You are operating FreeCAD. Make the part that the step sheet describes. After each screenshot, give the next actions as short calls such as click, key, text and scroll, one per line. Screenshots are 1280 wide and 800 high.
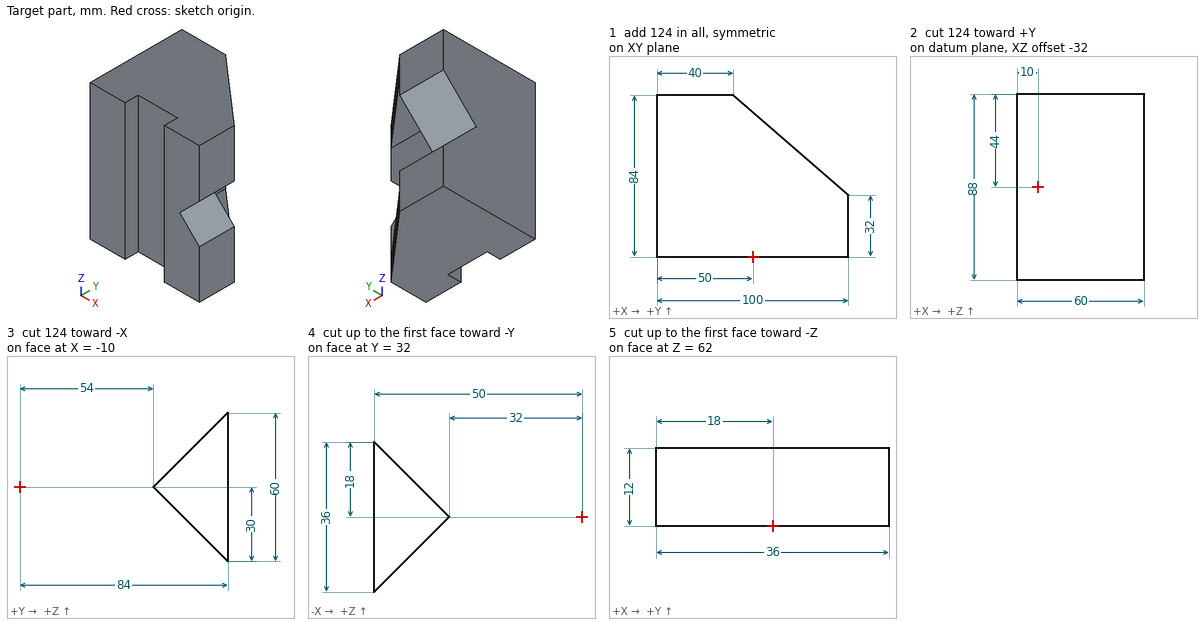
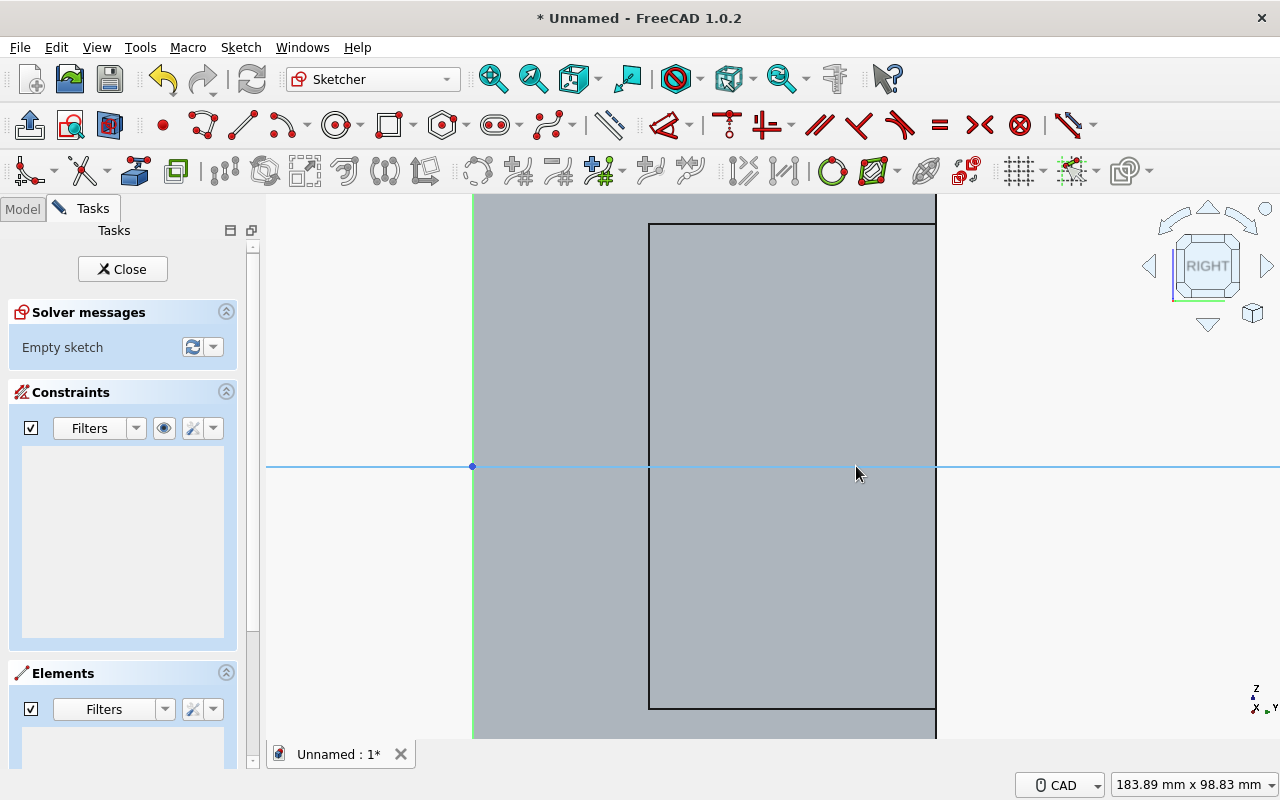
click(204, 126)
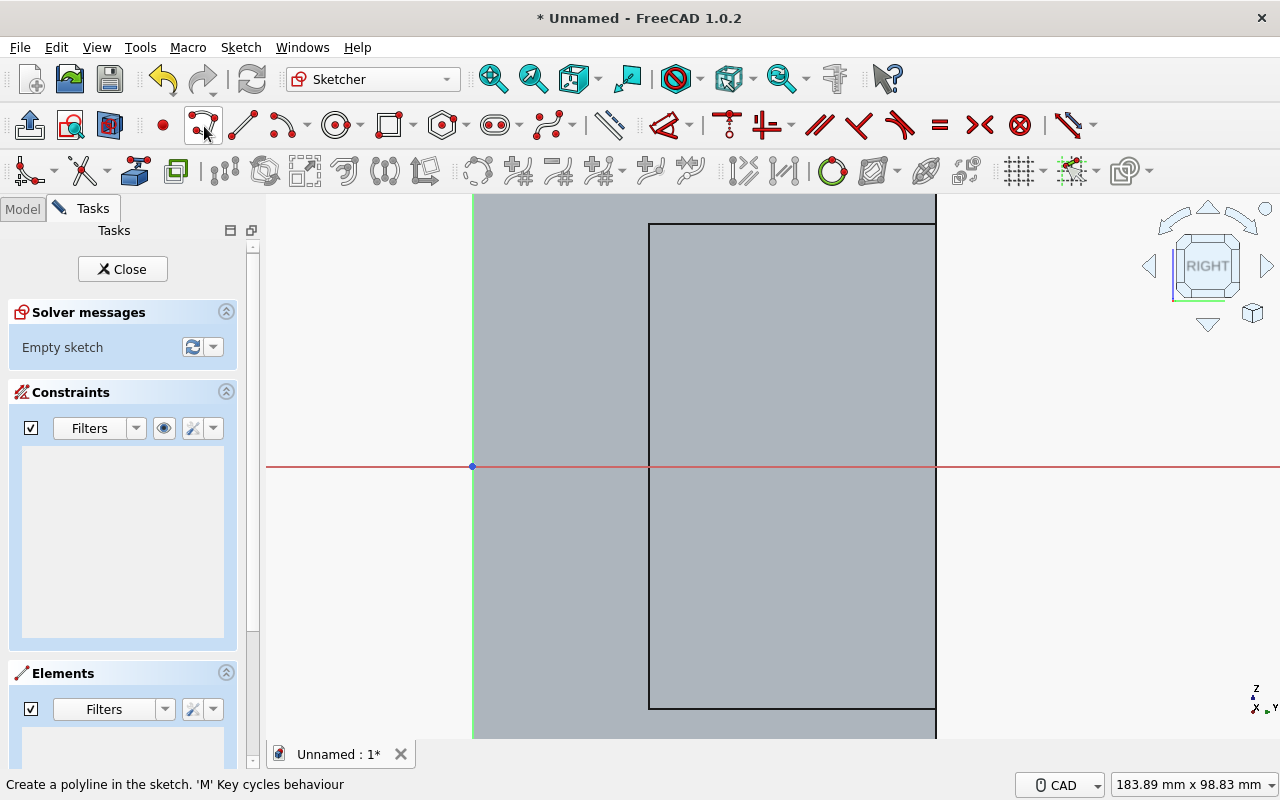
click(770, 466)
click(936, 632)
click(936, 301)
click(770, 466)
key(Escape)
key(Escape)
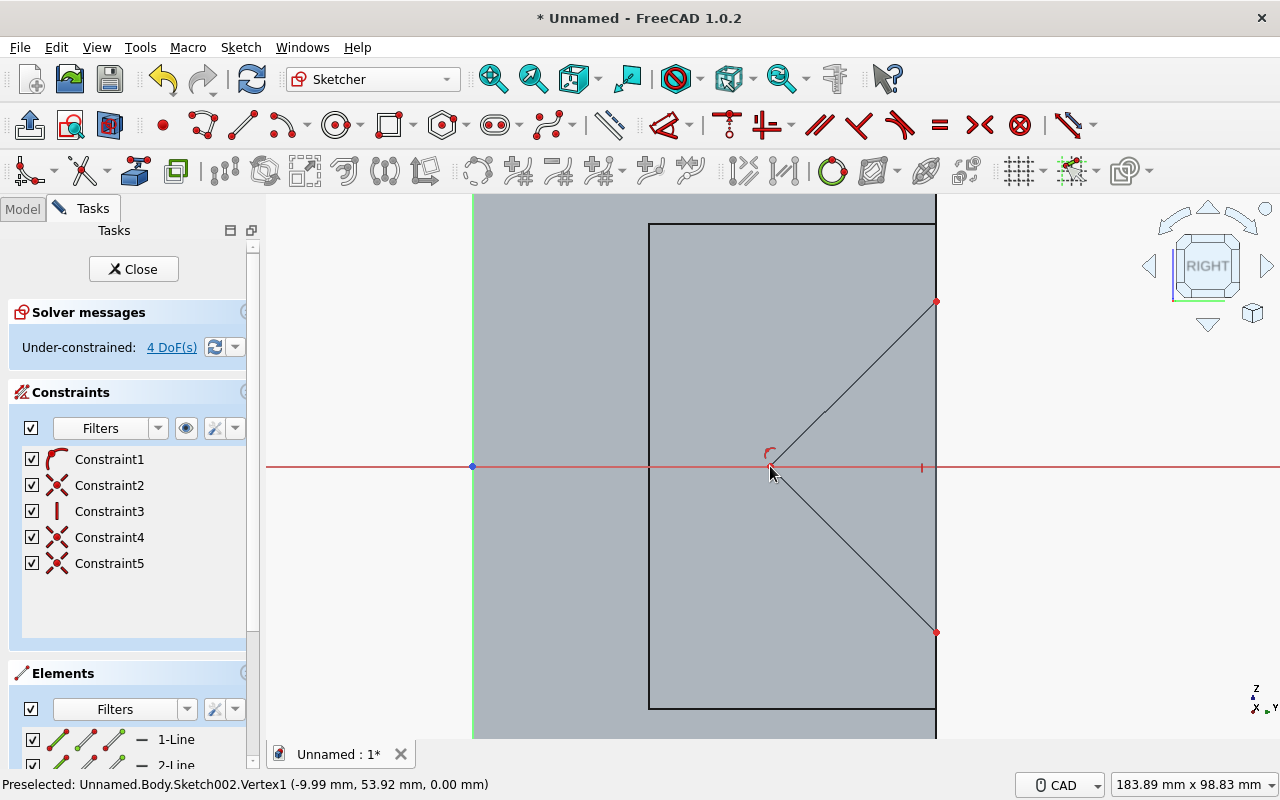
click(664, 126)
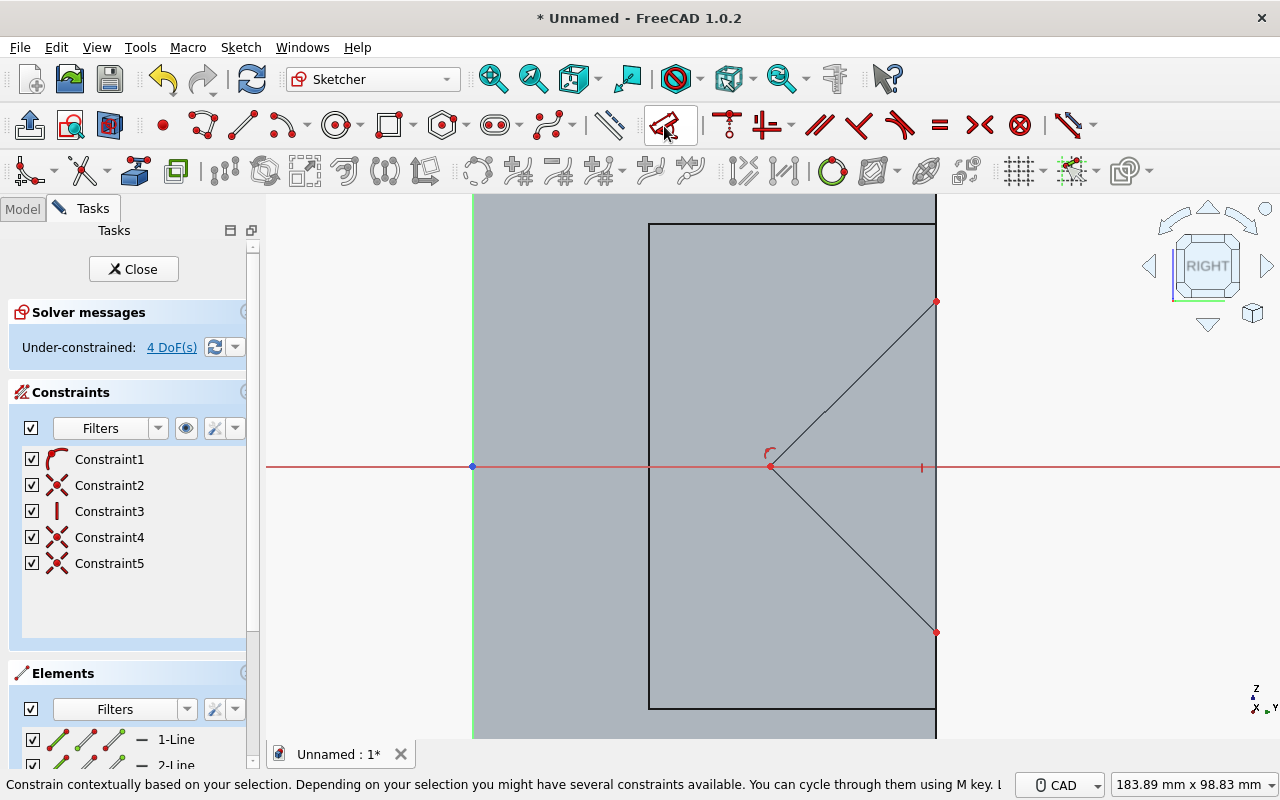
click(936, 534)
click(970, 391)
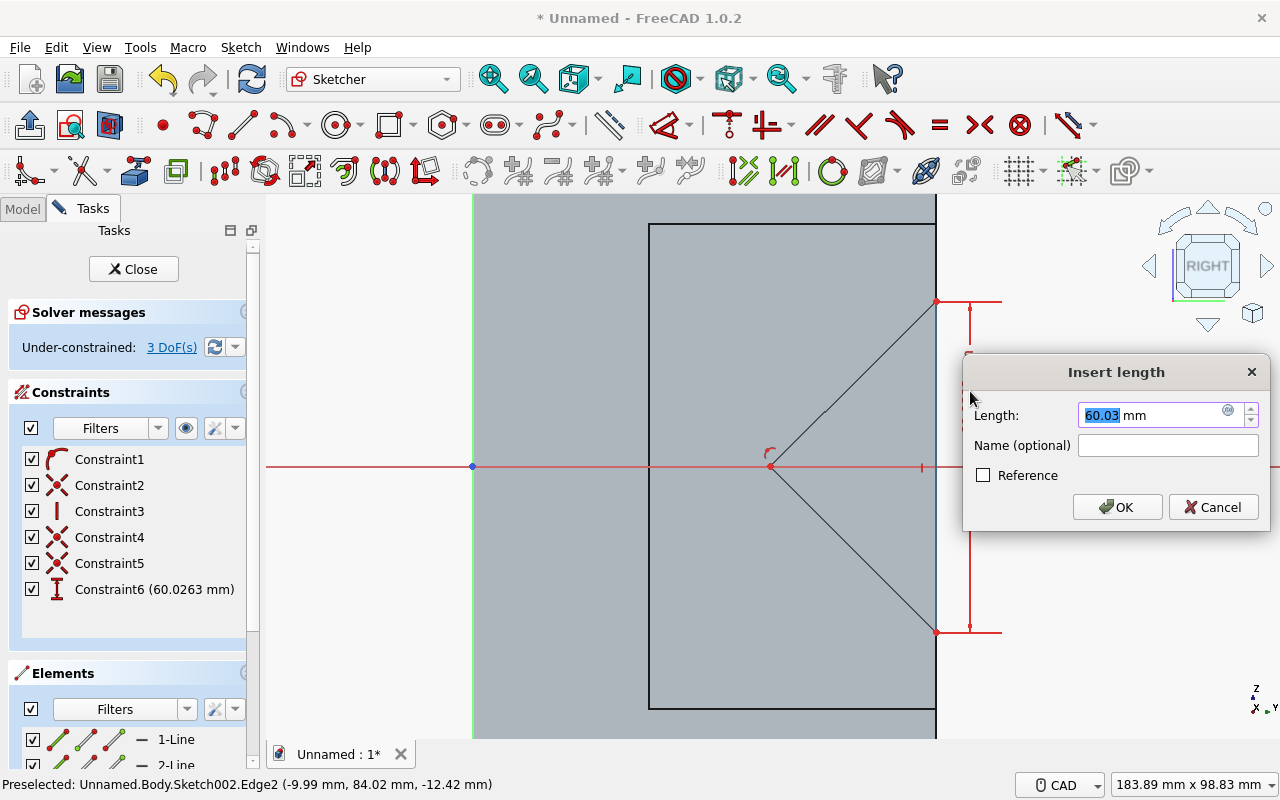
text(60)
key(Return)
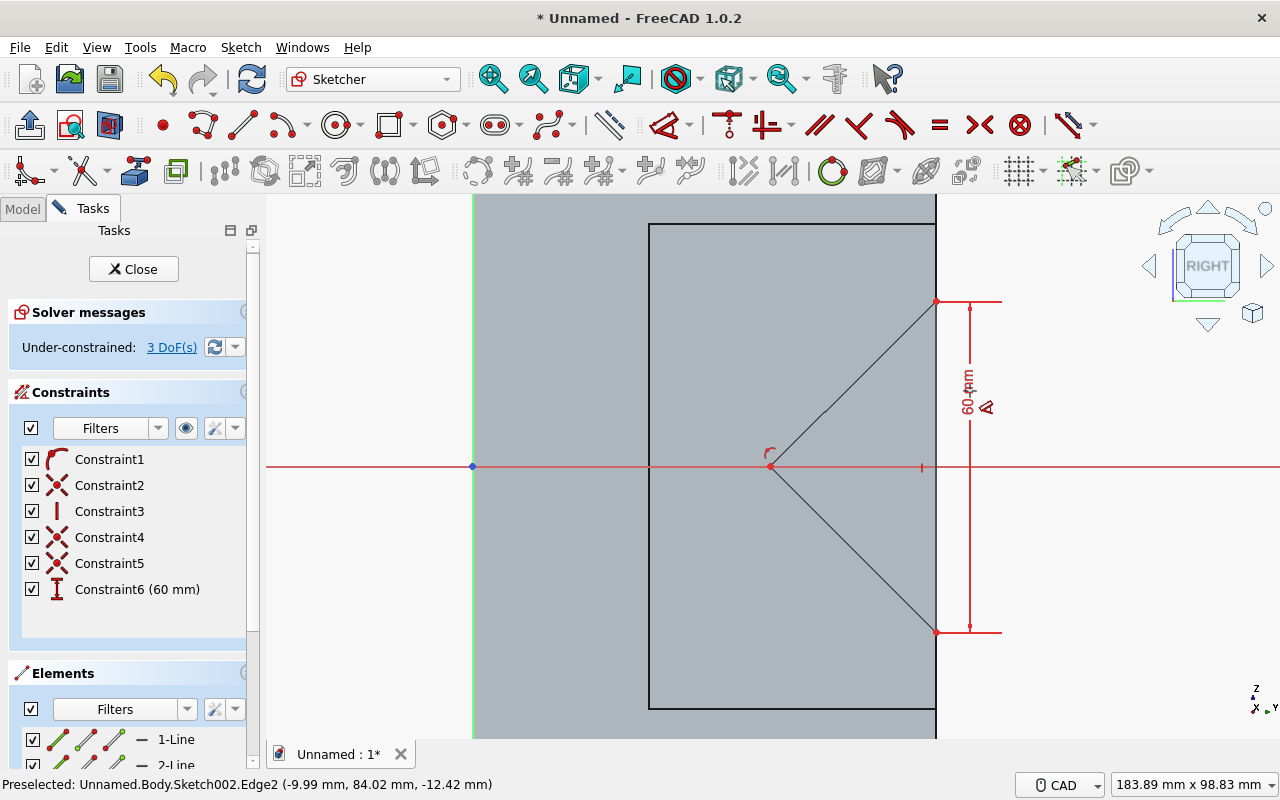
click(770, 466)
click(621, 500)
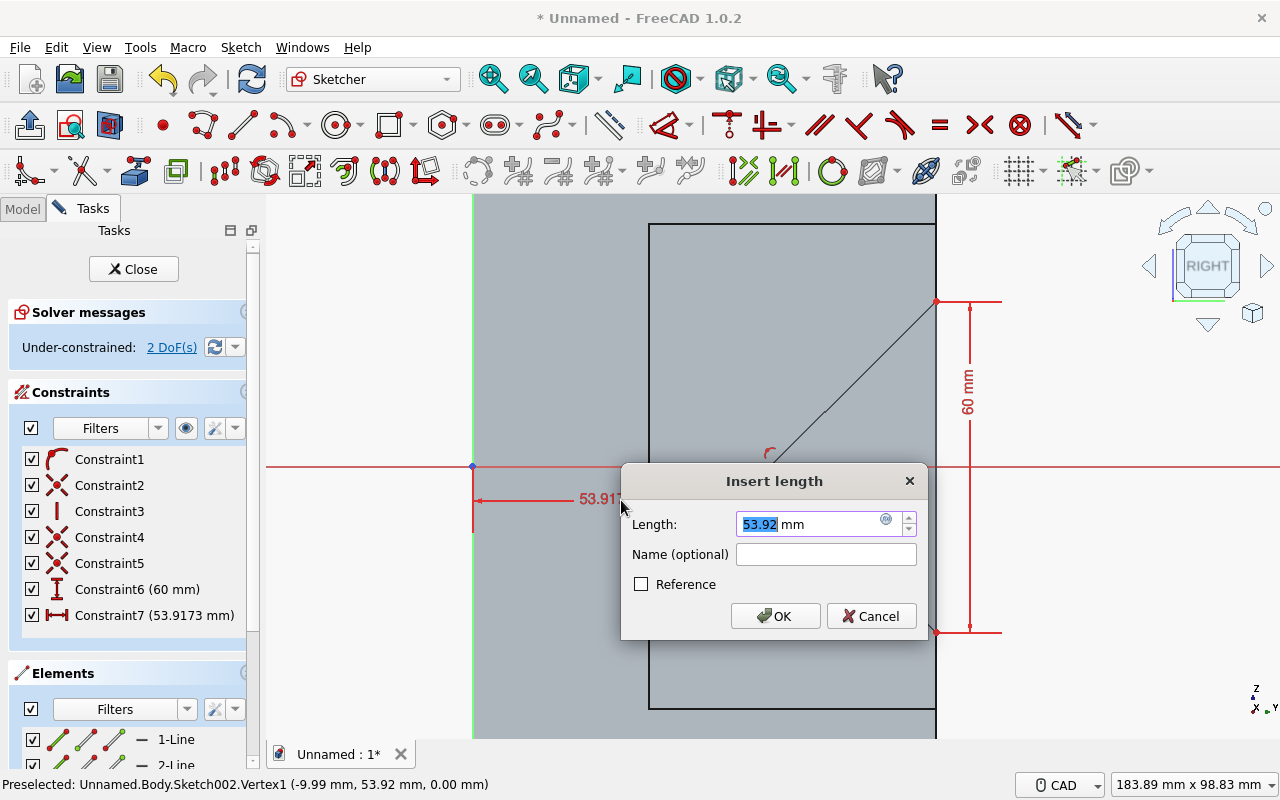
text(54)
key(Return)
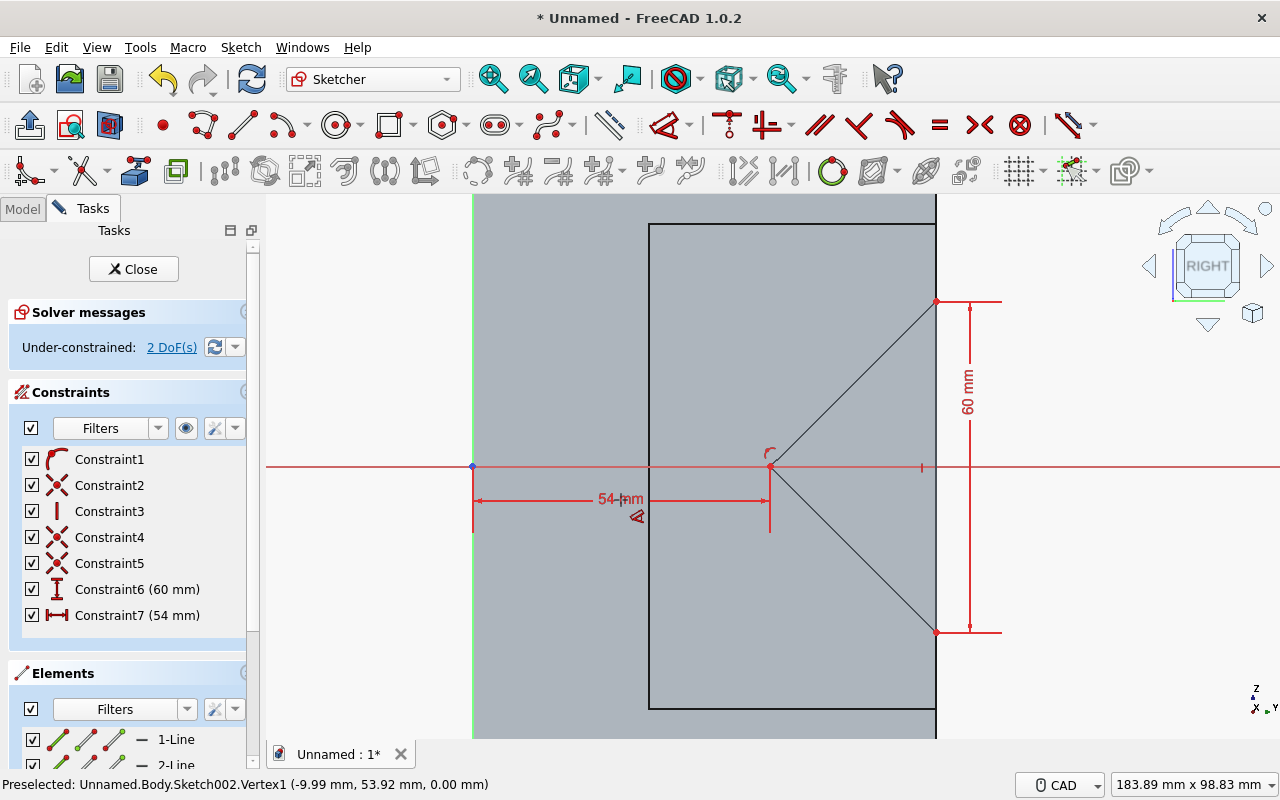
click(936, 633)
click(704, 667)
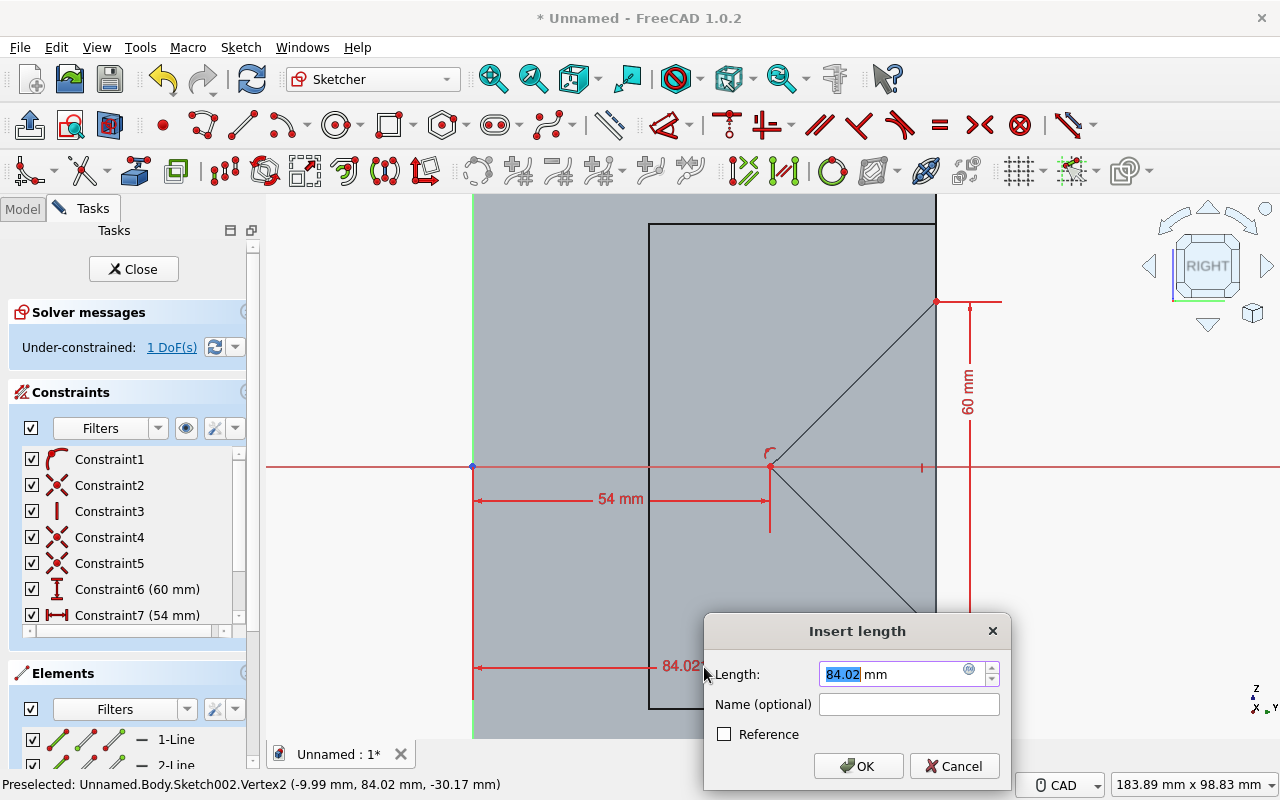
text(84)
key(Return)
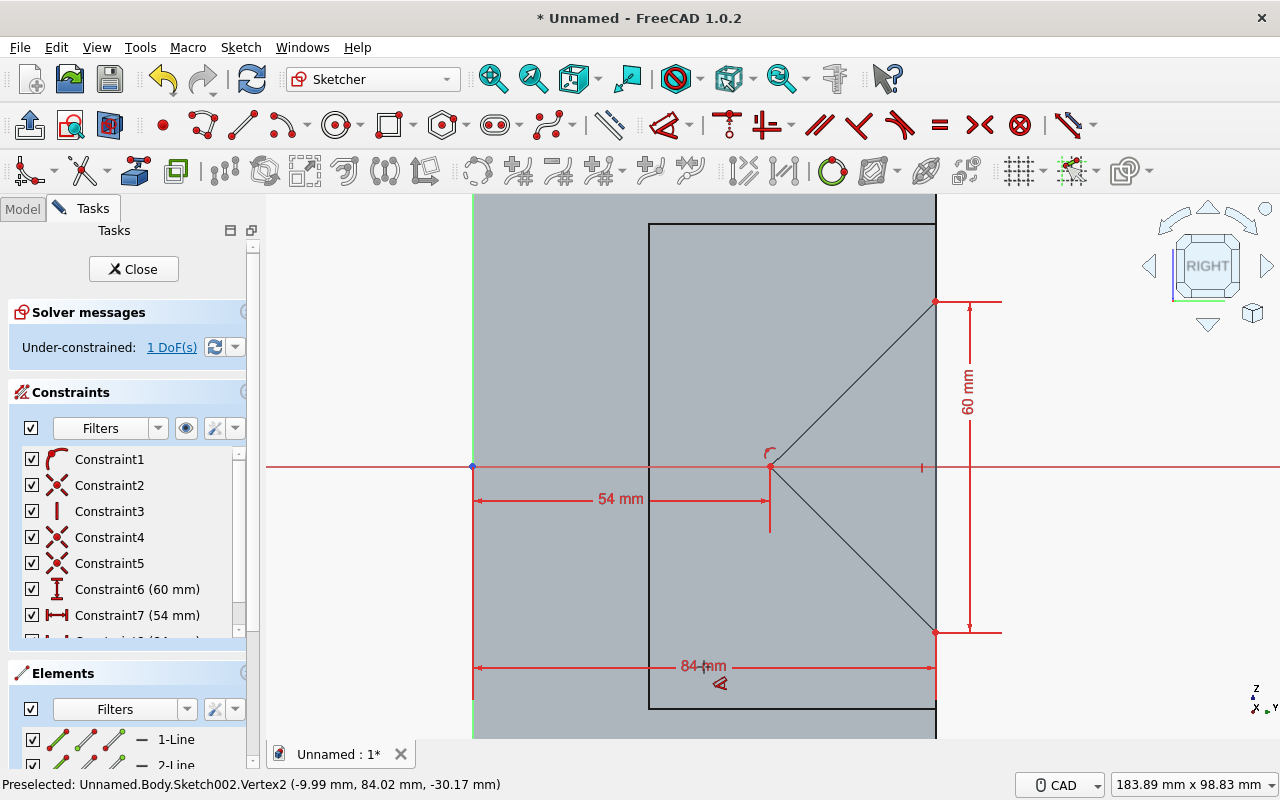
click(936, 633)
click(970, 550)